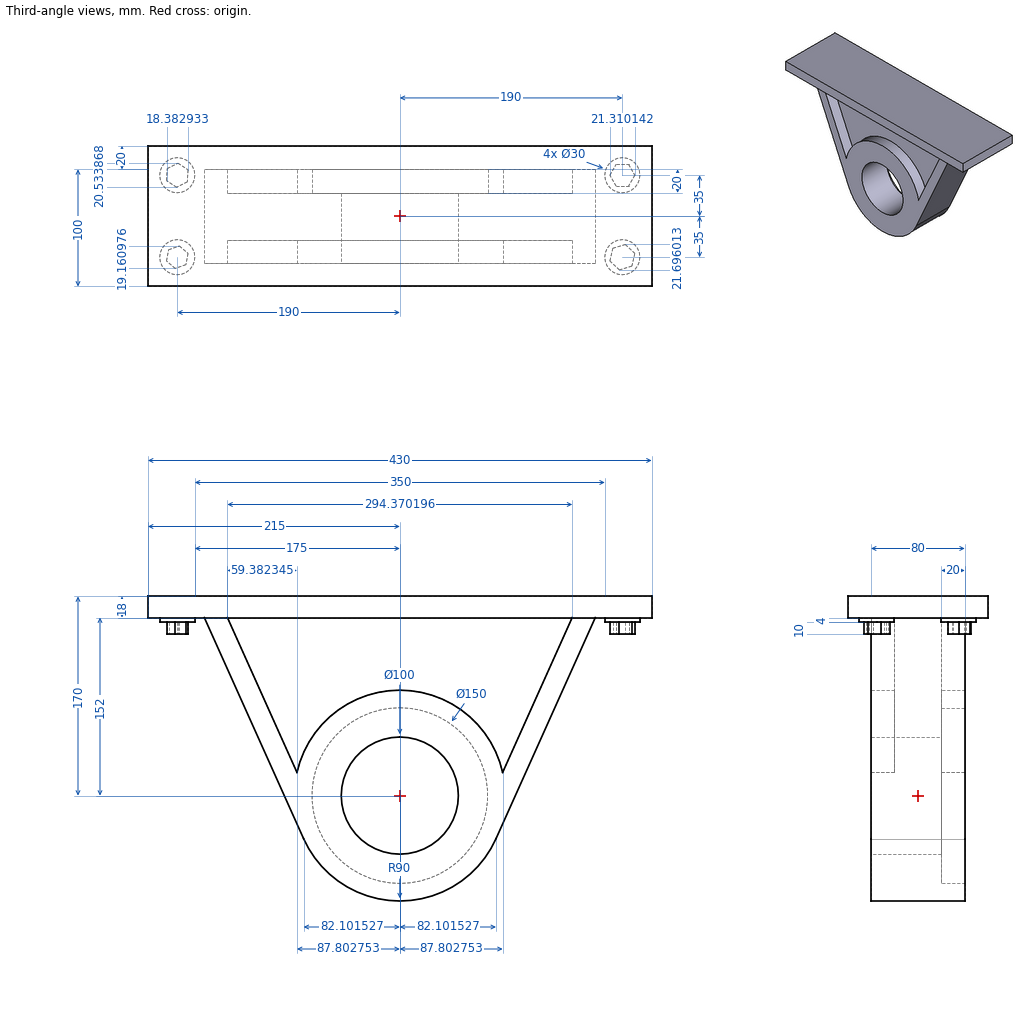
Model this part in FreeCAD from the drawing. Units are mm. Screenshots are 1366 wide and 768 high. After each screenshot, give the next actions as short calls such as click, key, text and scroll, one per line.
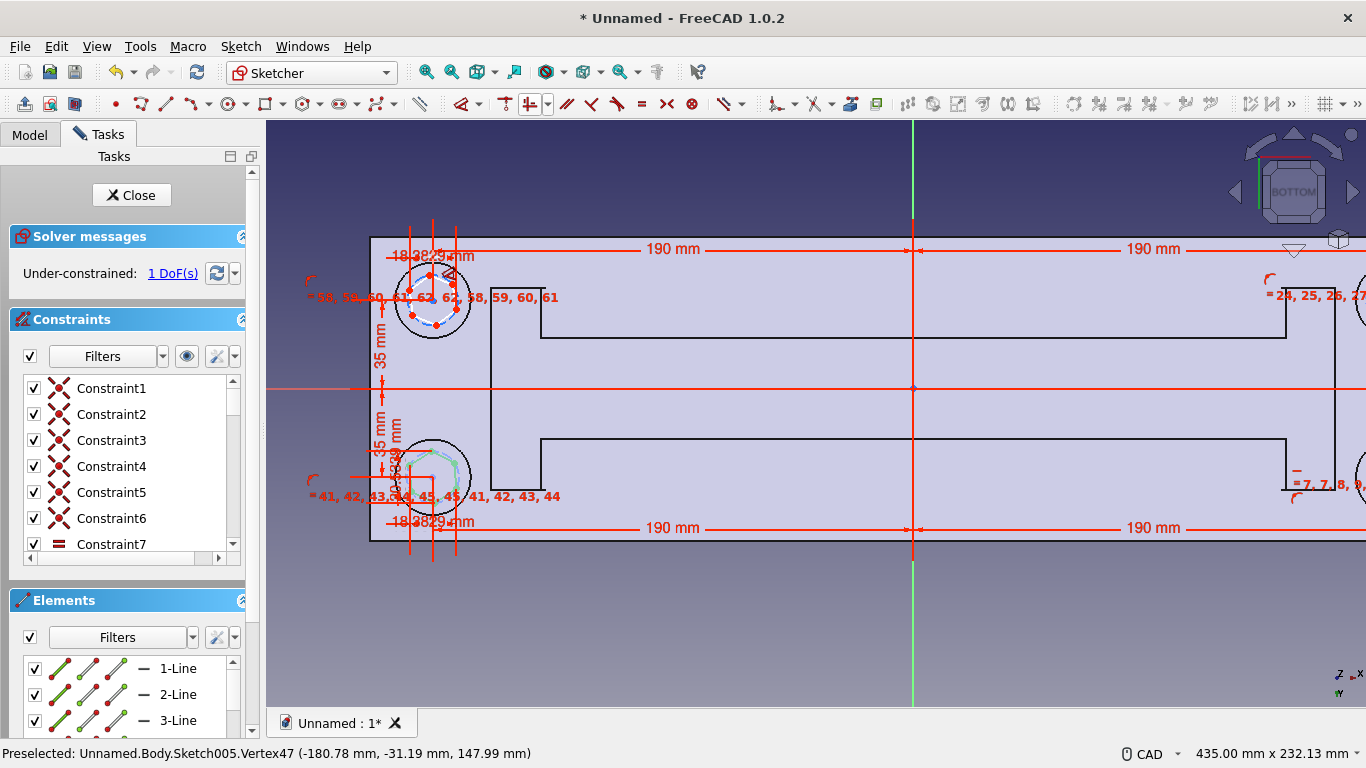
click(436, 325)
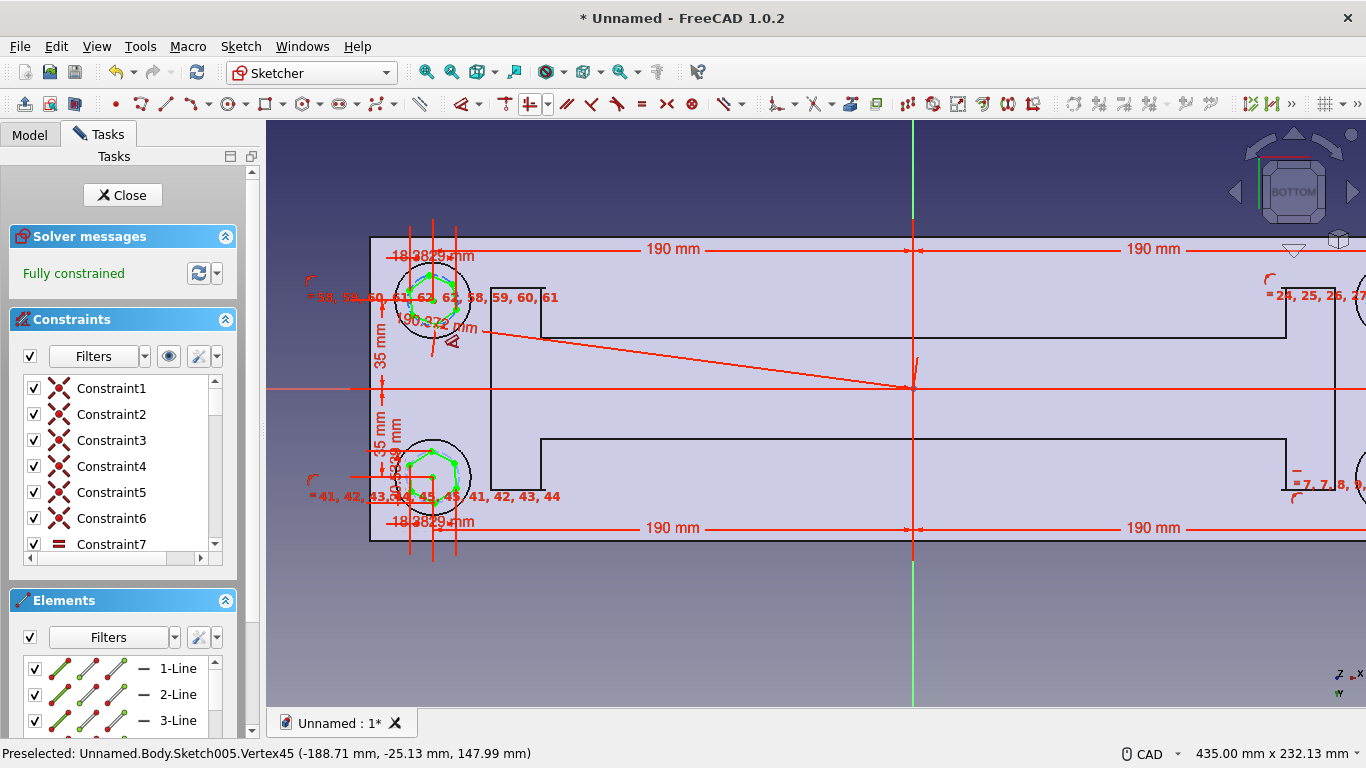
click(430, 275)
click(396, 289)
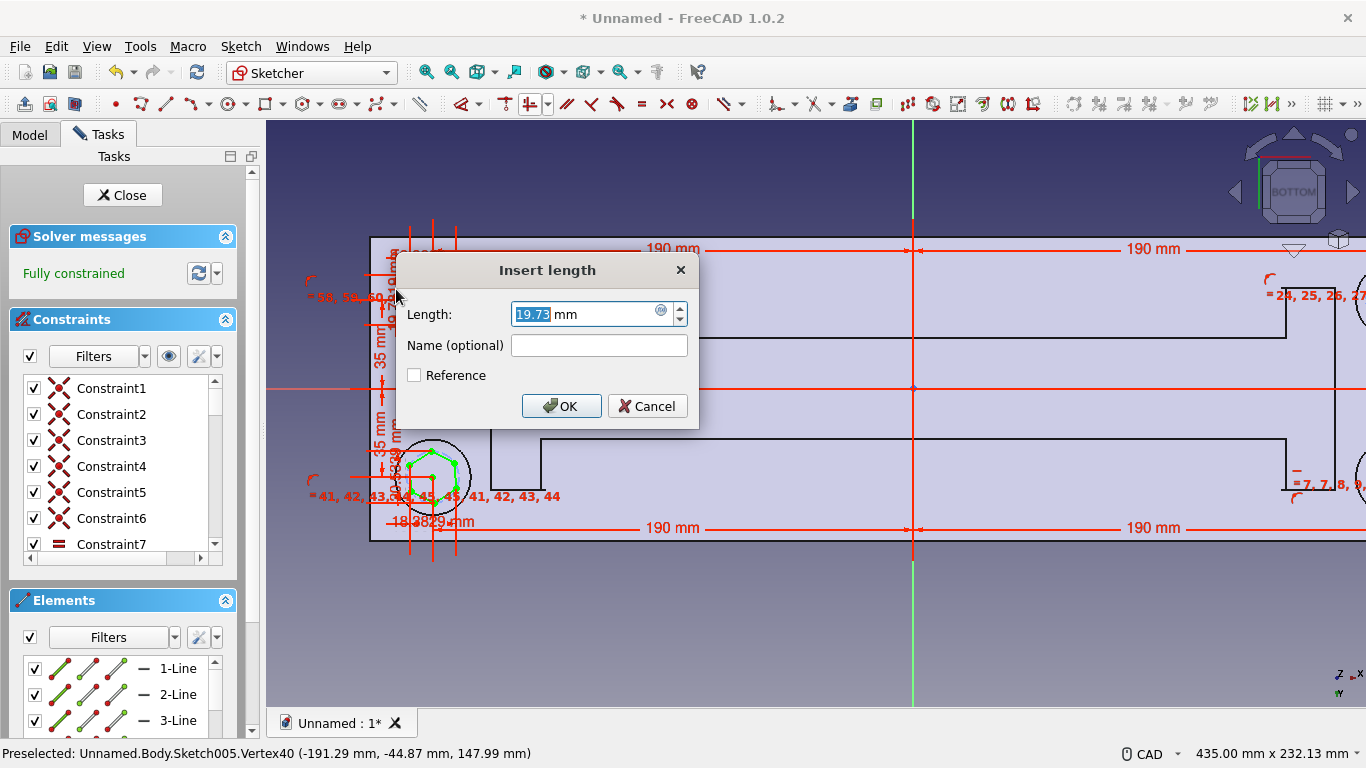
text(19.160976)
key(Return)
key(Escape)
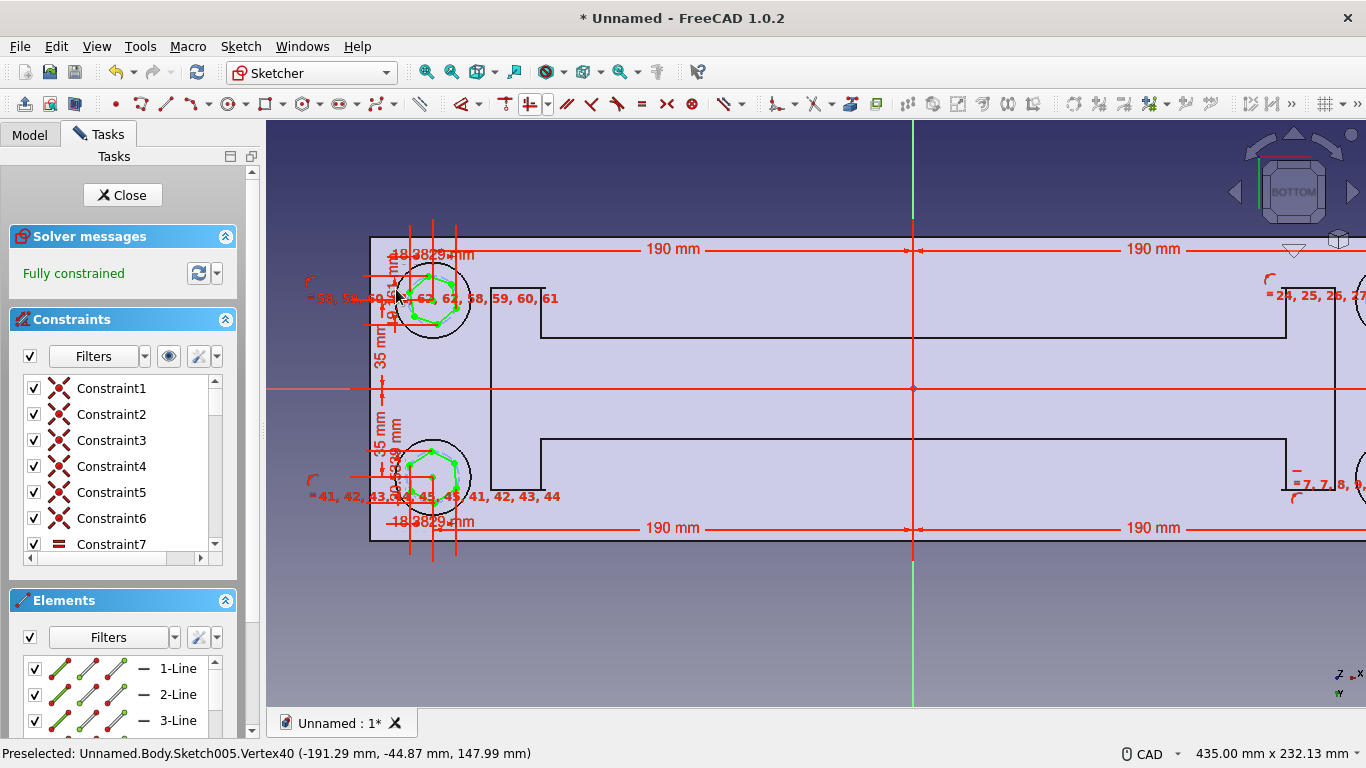
click(123, 195)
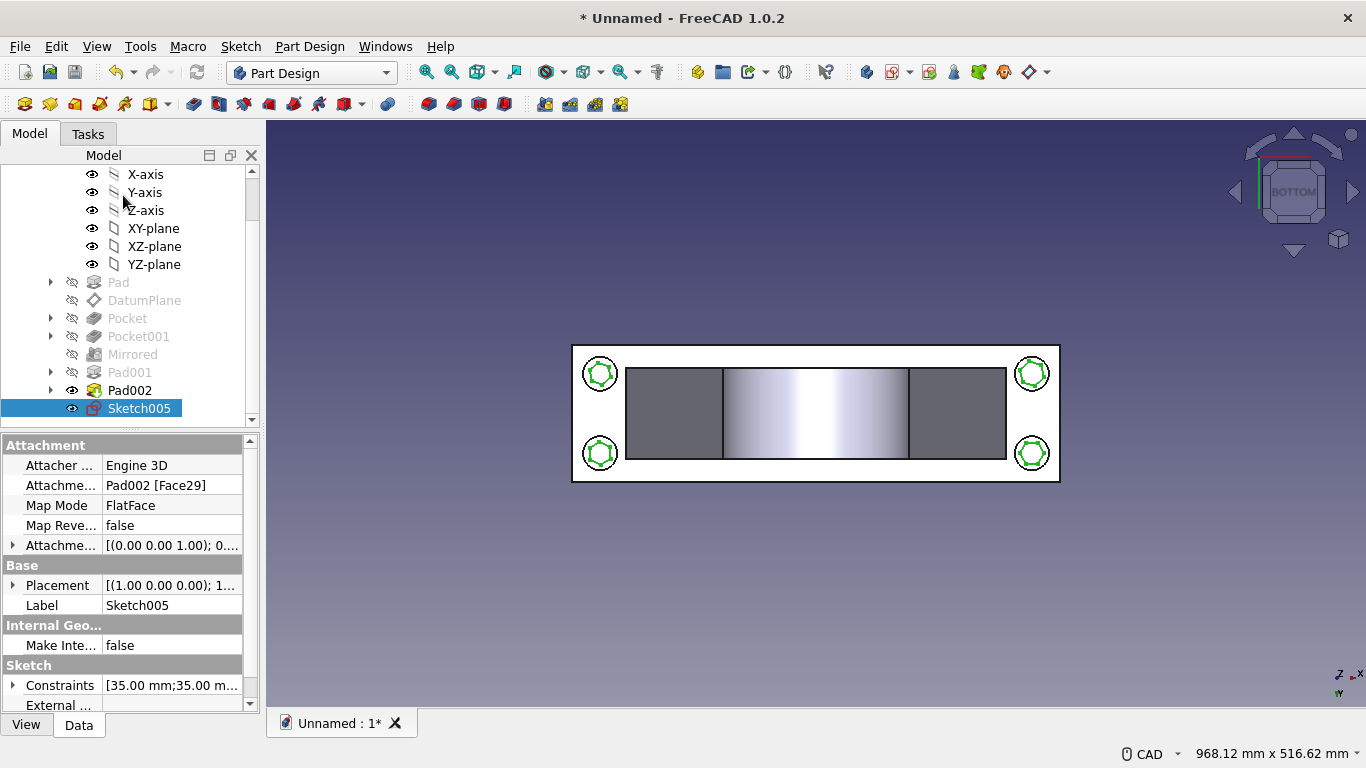
click(25, 104)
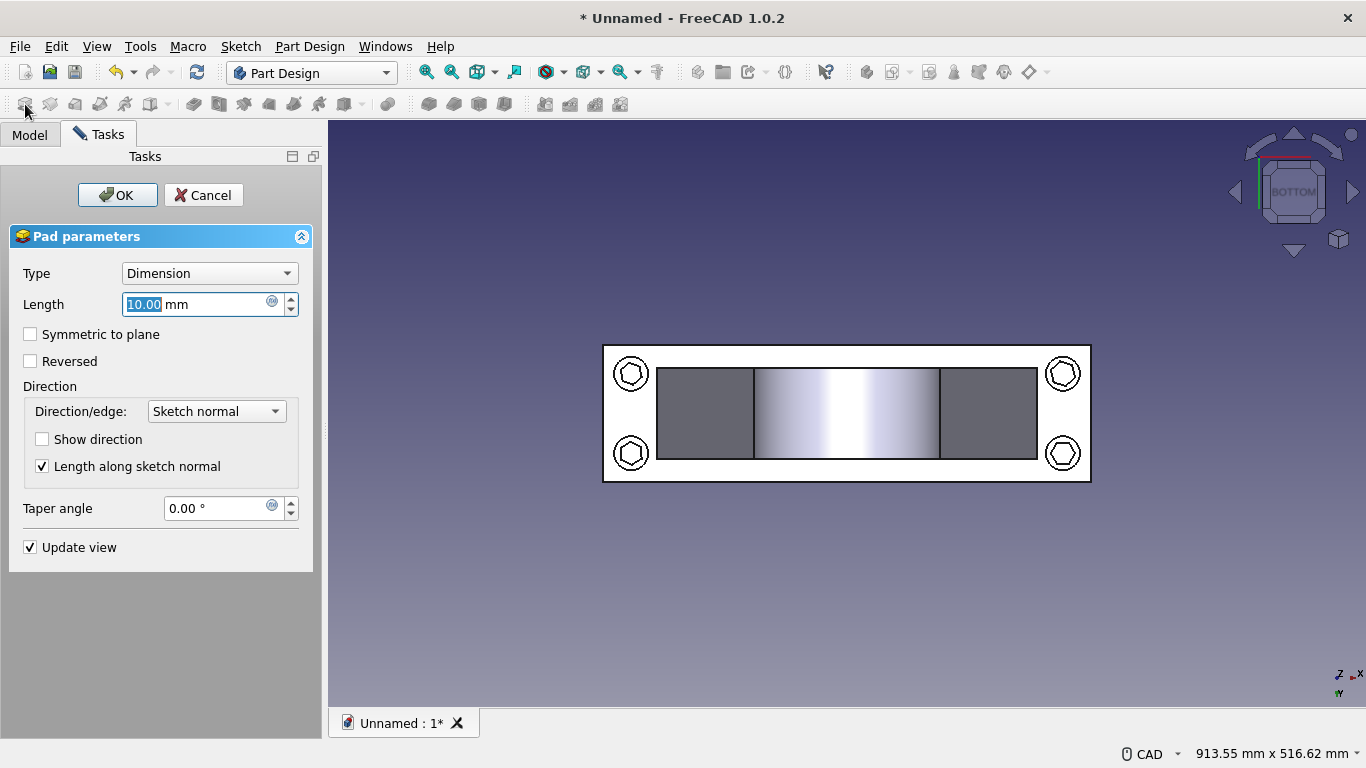
text(10)
key(Tab)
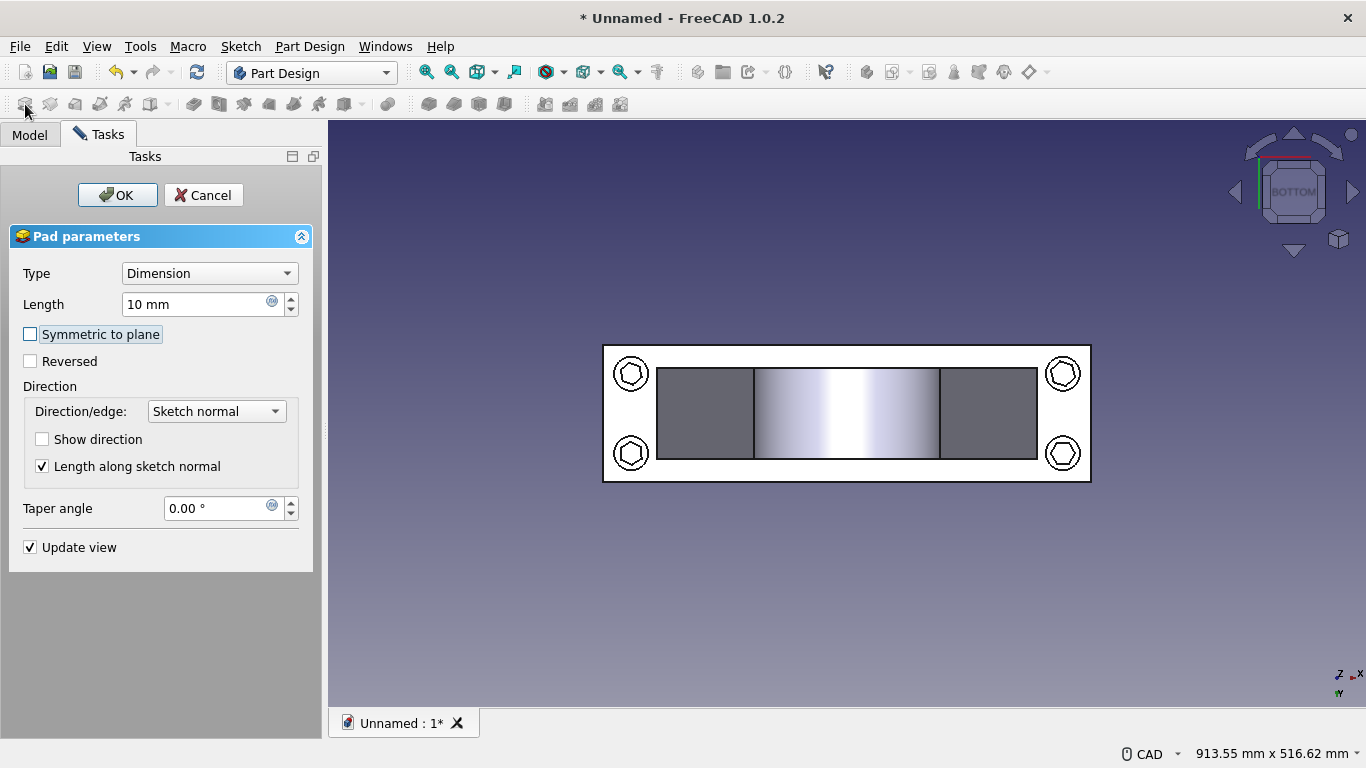
click(118, 195)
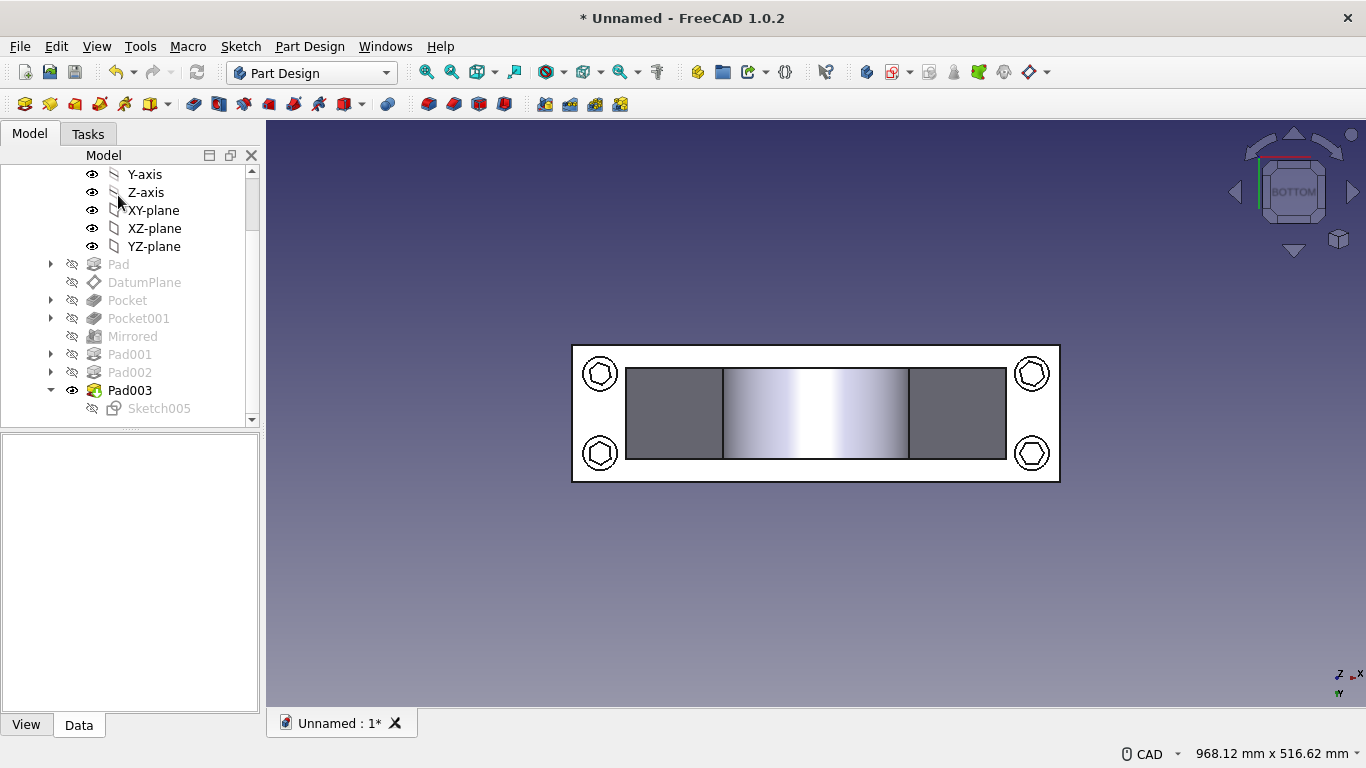
key(0)